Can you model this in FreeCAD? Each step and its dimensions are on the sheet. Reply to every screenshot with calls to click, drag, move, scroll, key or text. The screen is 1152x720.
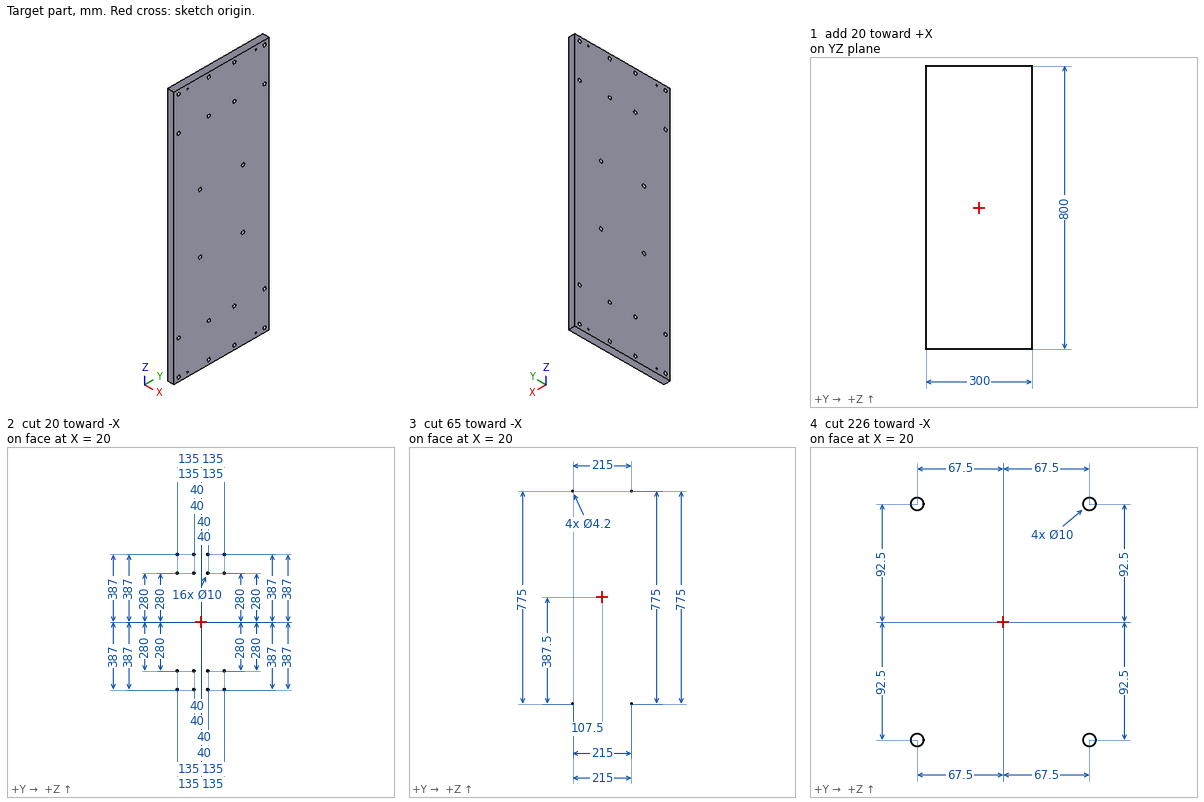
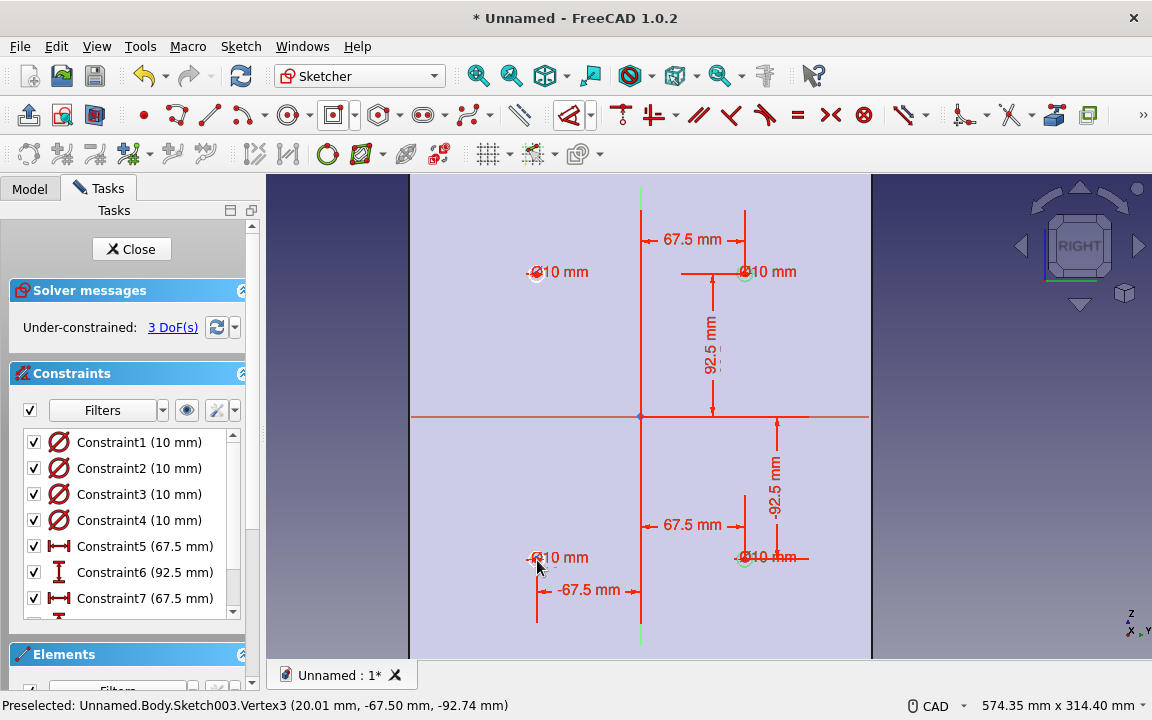
click(537, 560)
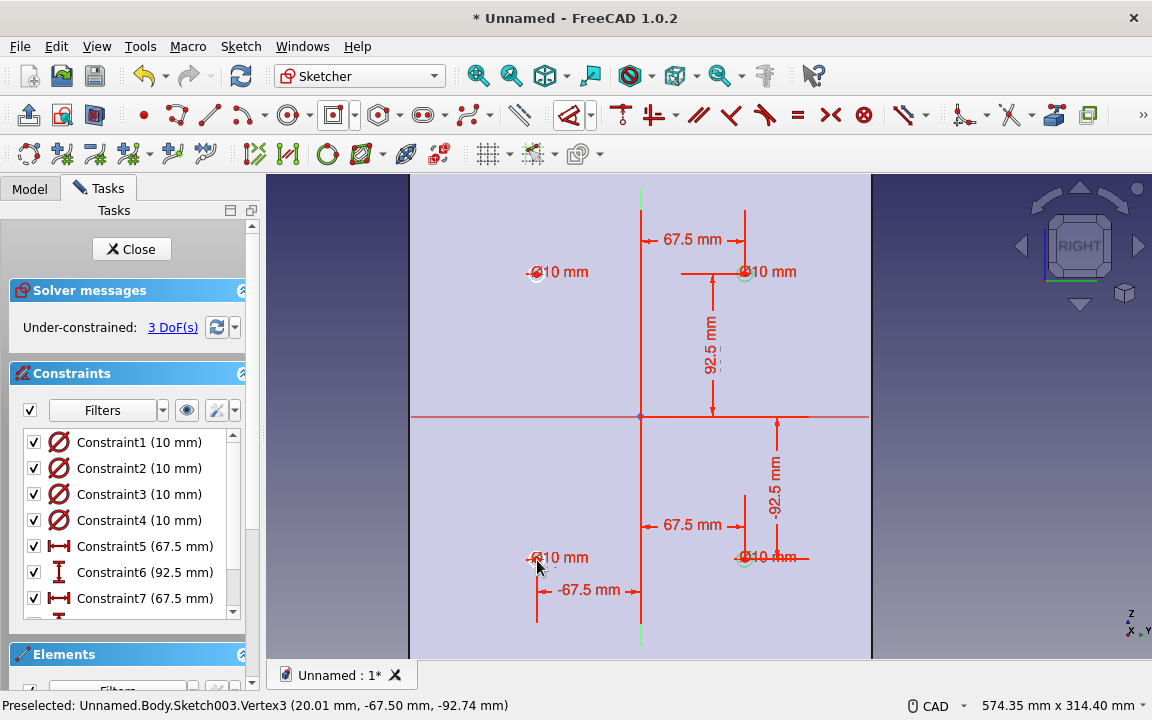
key(i)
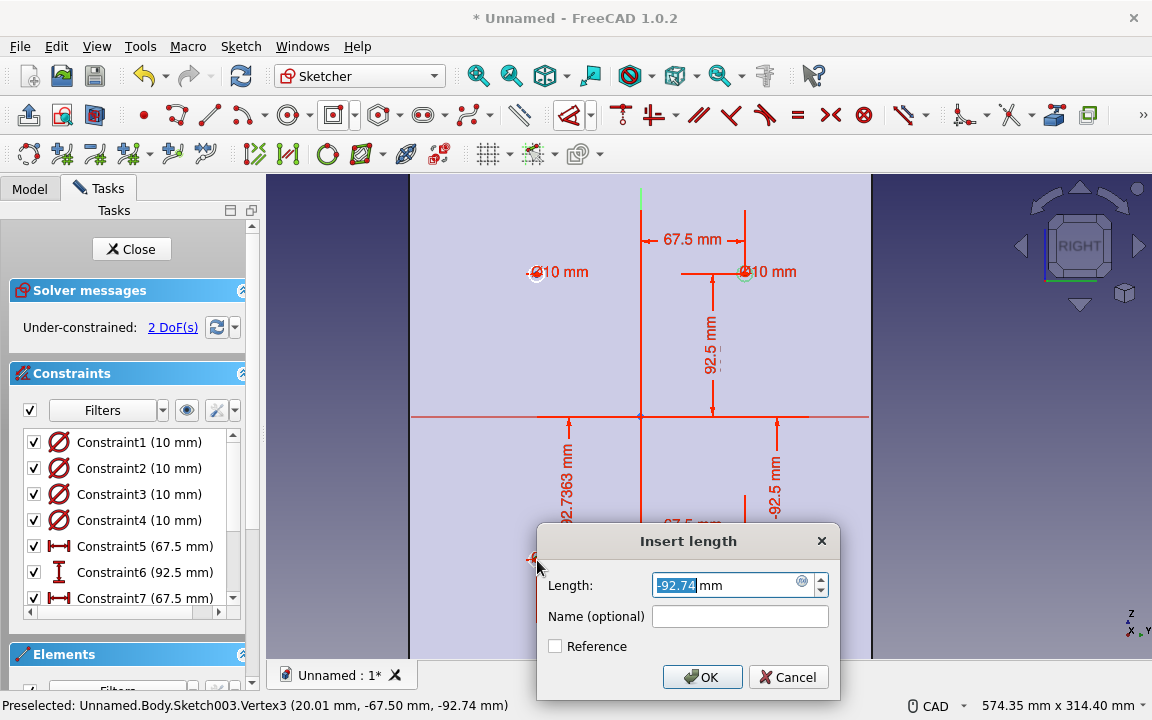
text(-92.5)
key(Return)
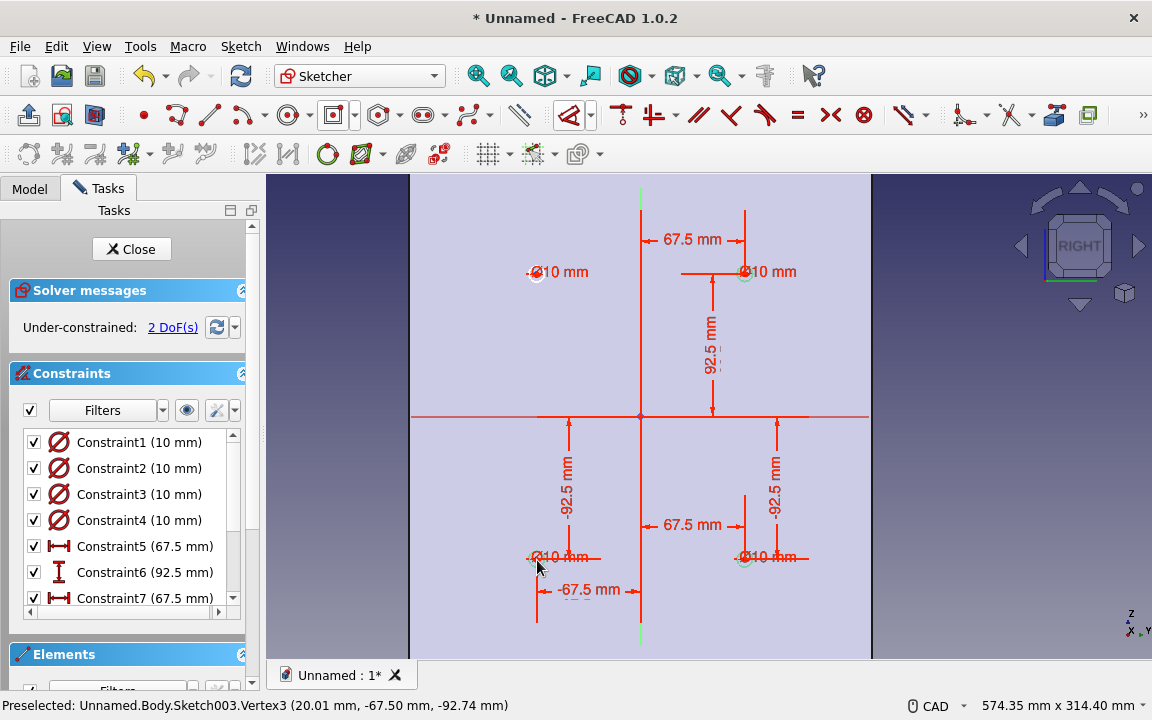
click(537, 274)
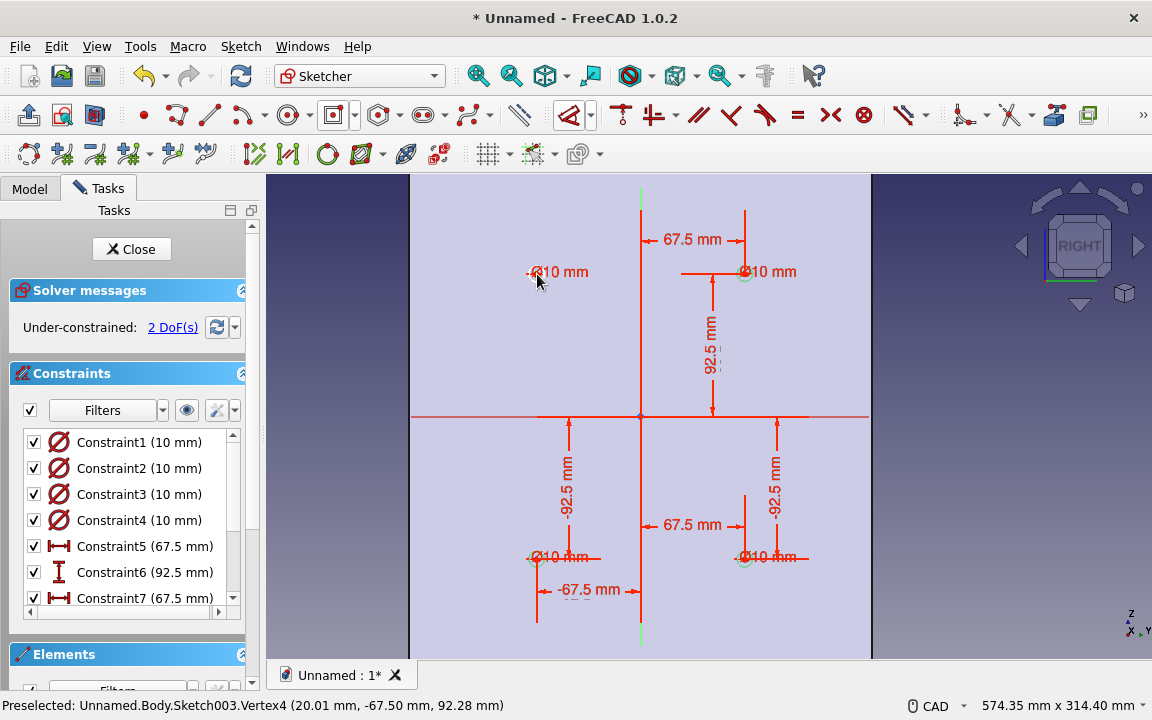
key(l)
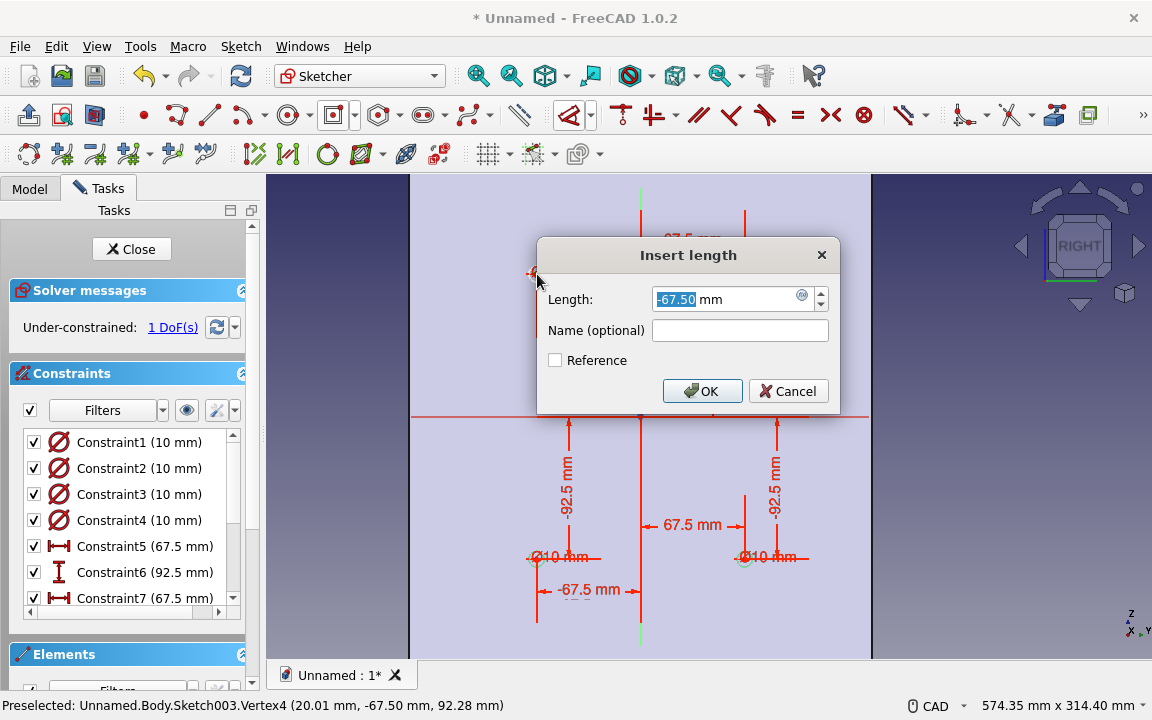
text(-67.5)
key(Return)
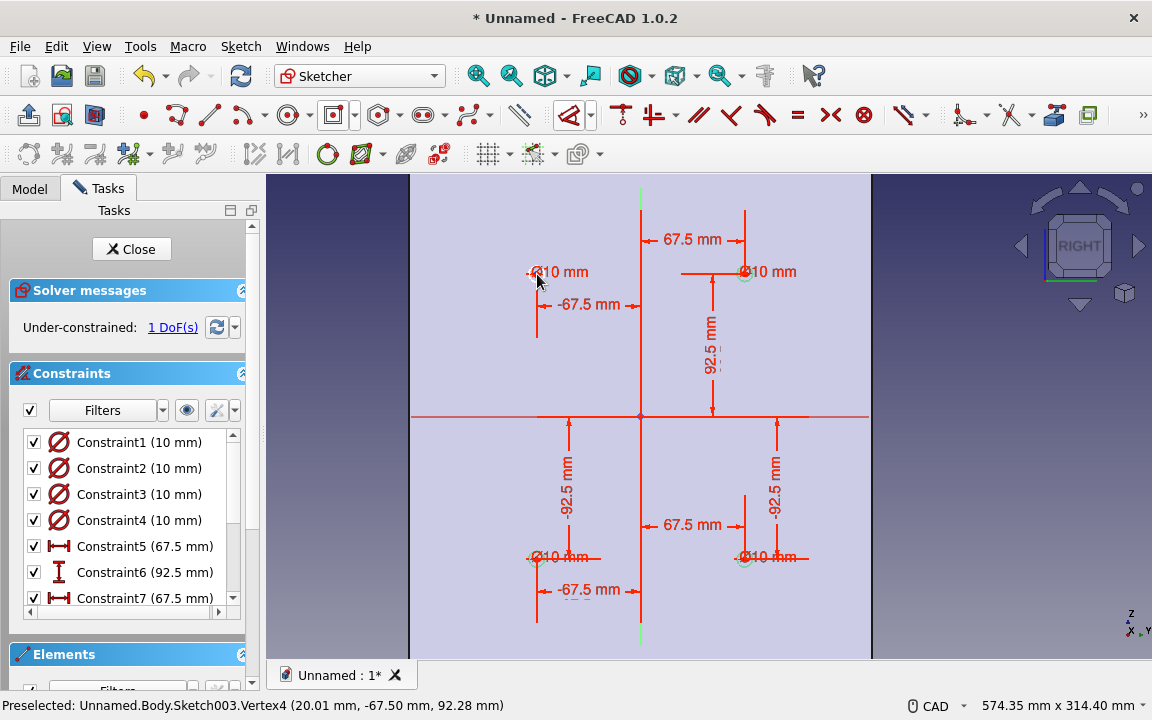
click(537, 274)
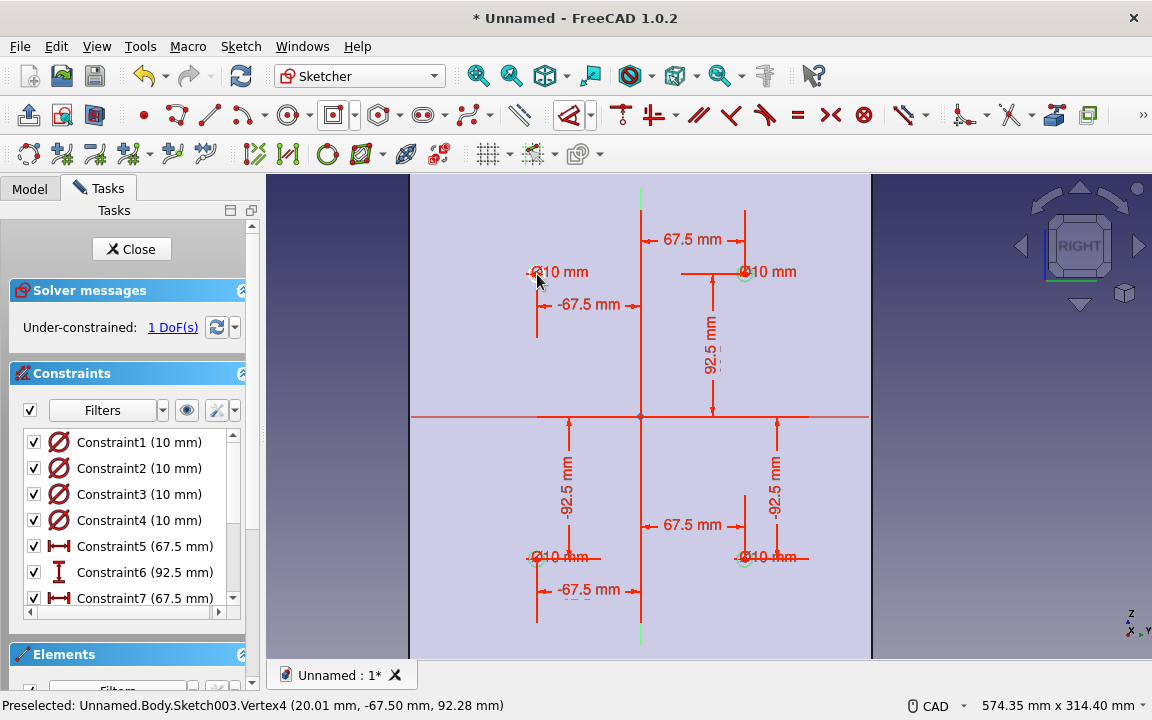
click(590, 116)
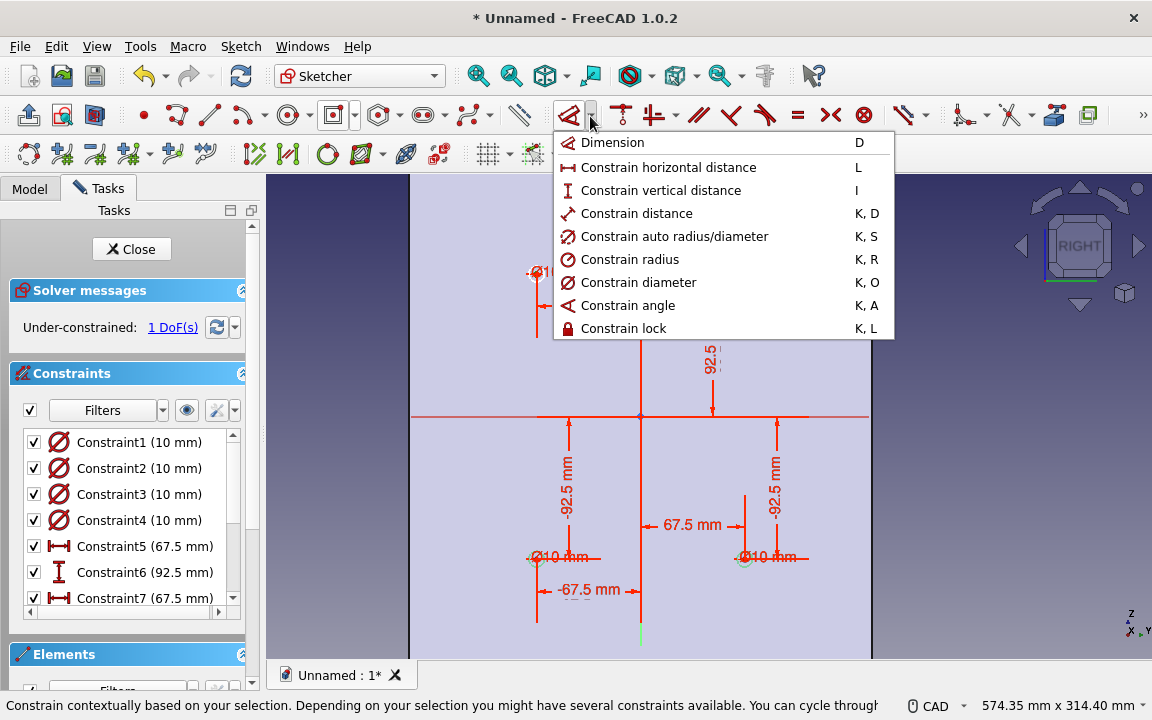
click(724, 190)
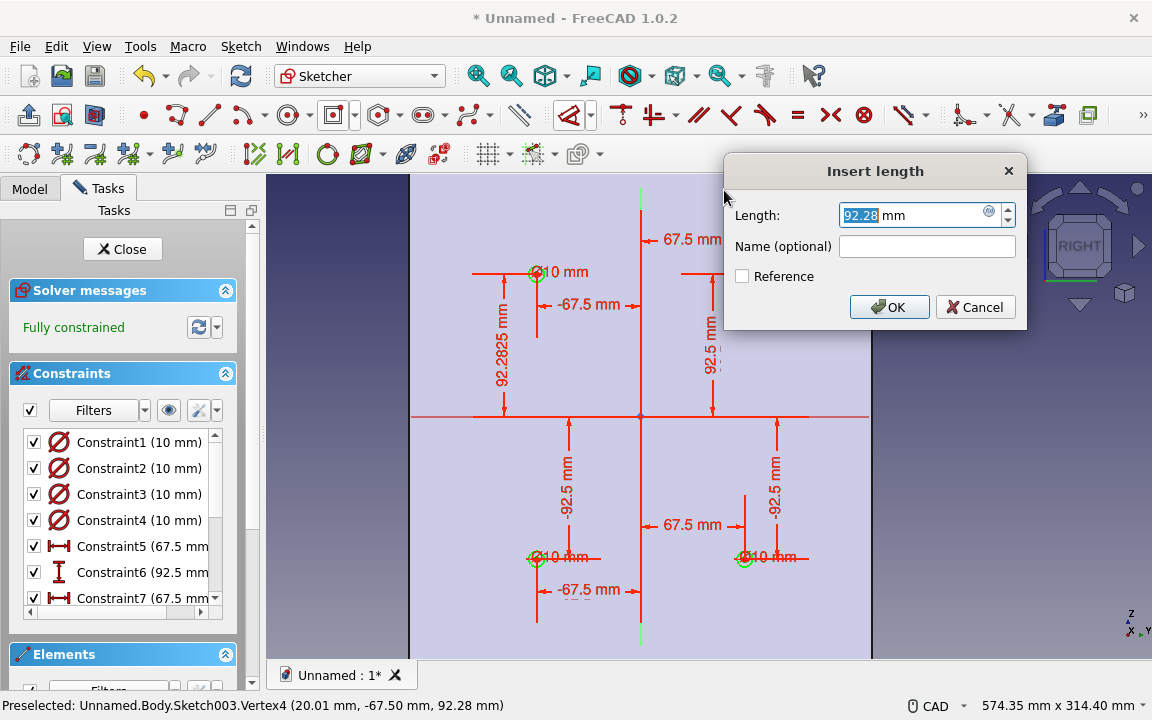
text(92.5)
key(Return)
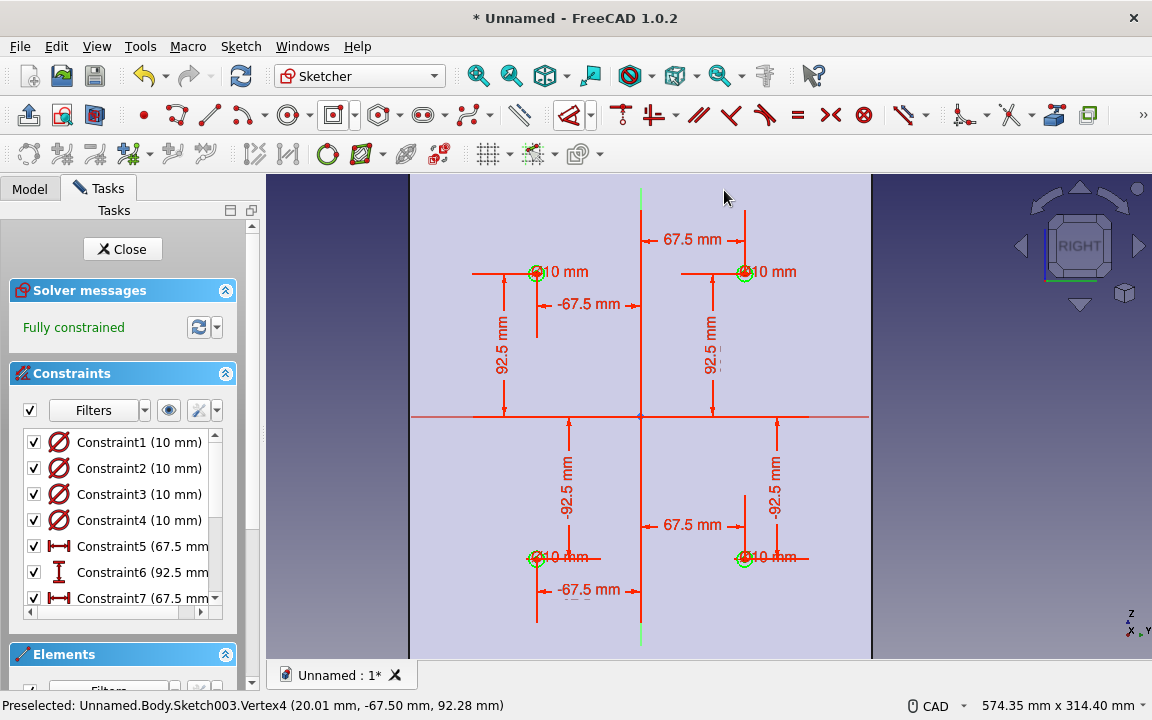
click(123, 249)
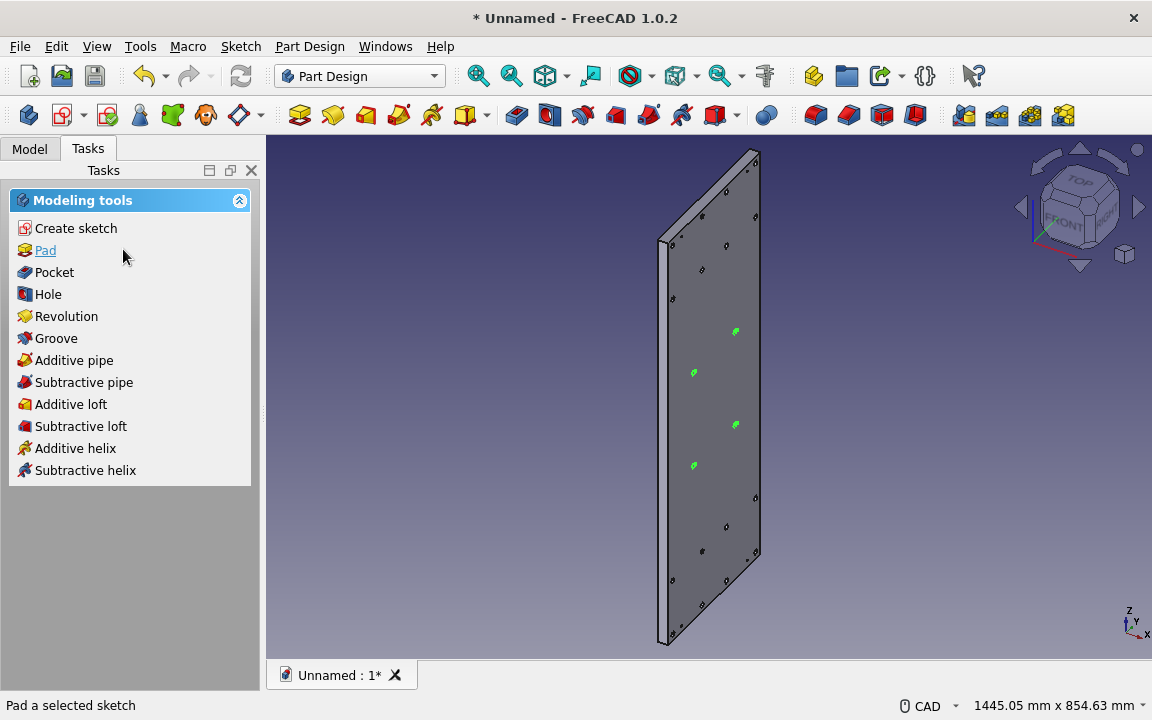
click(517, 116)